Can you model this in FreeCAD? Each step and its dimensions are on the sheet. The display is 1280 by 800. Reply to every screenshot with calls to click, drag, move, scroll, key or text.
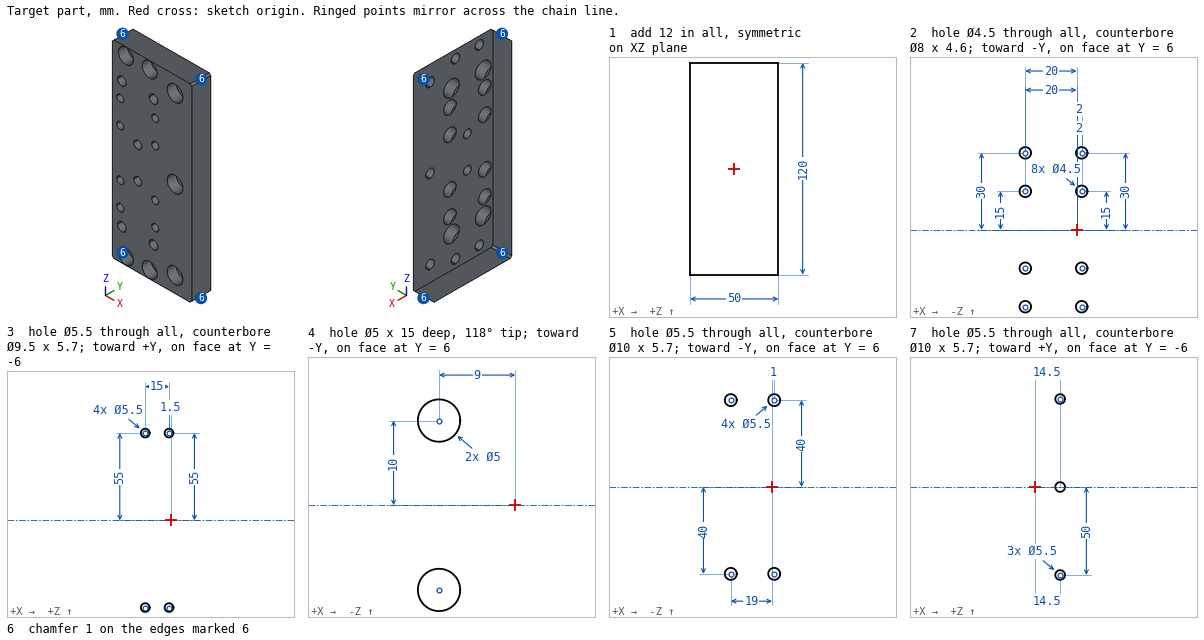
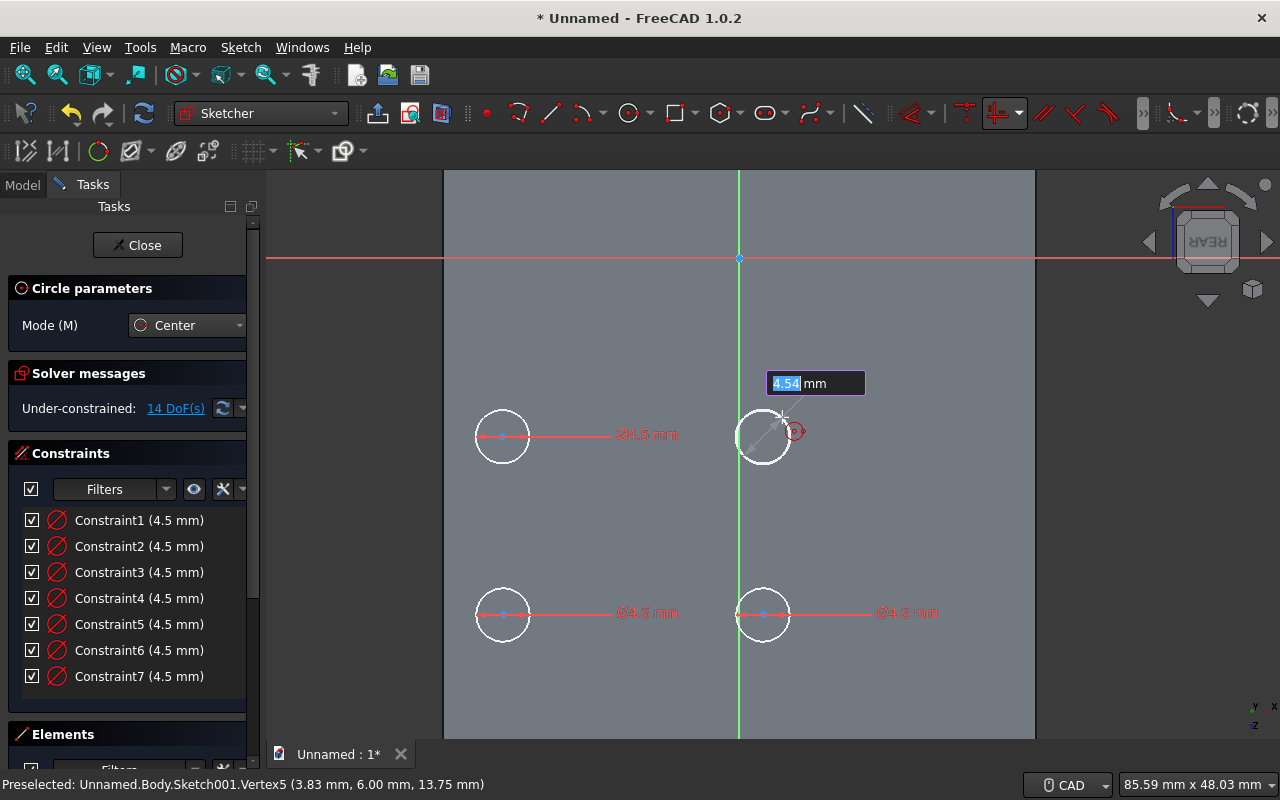
text(4.5)
key(Return)
key(Escape)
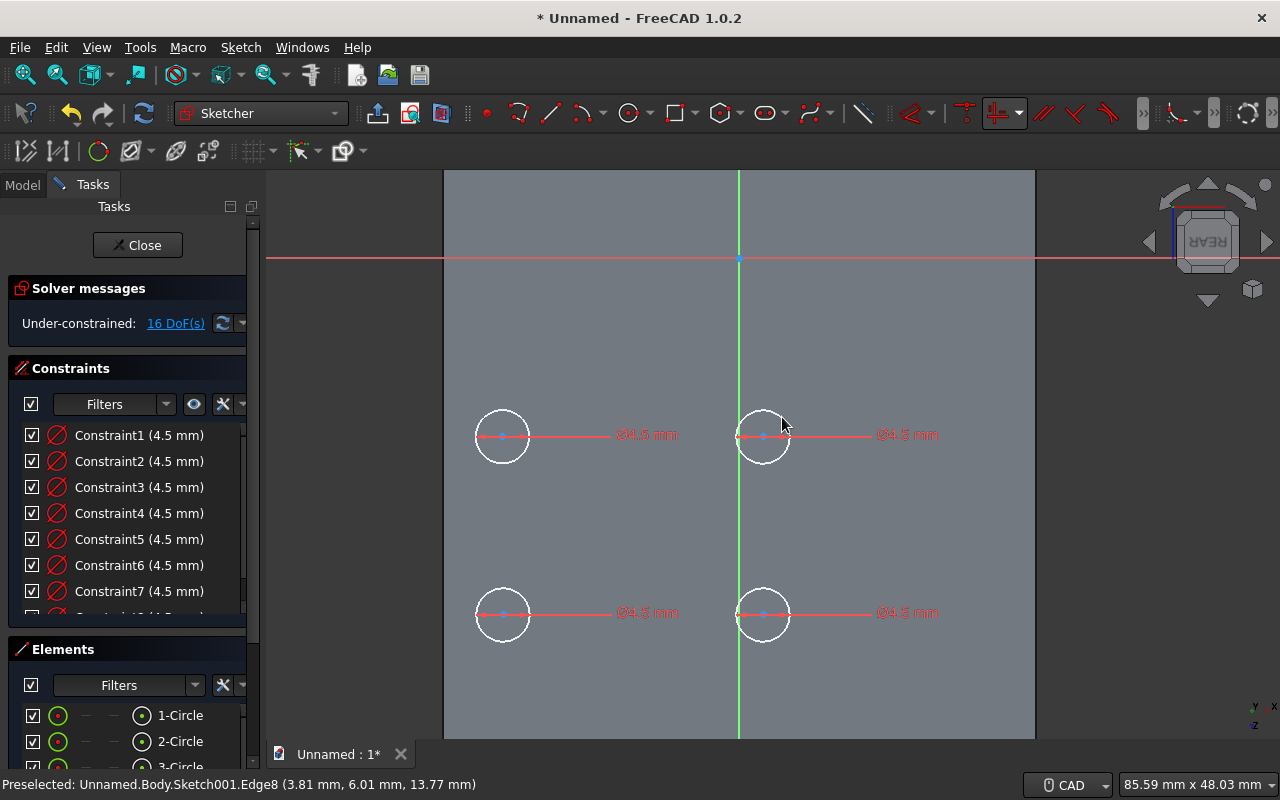
scroll(763, 615, down, 4)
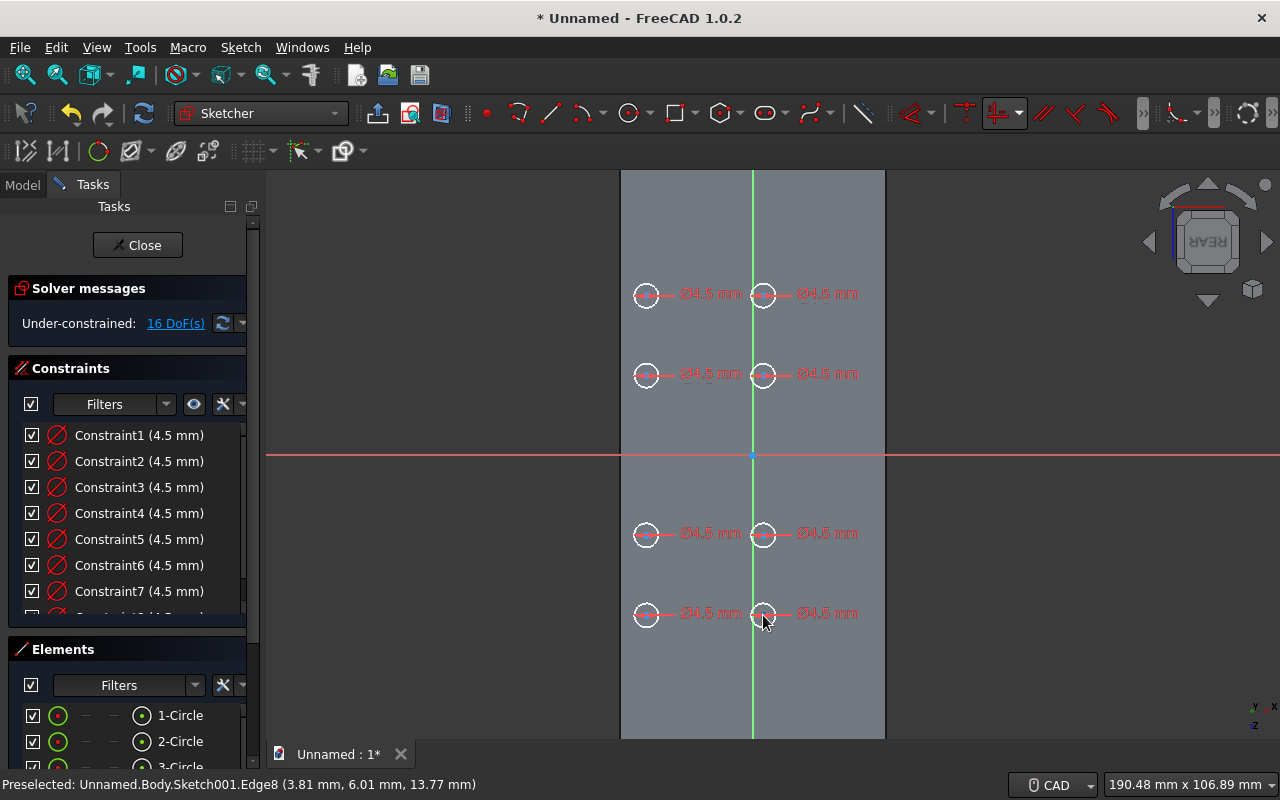
click(646, 376)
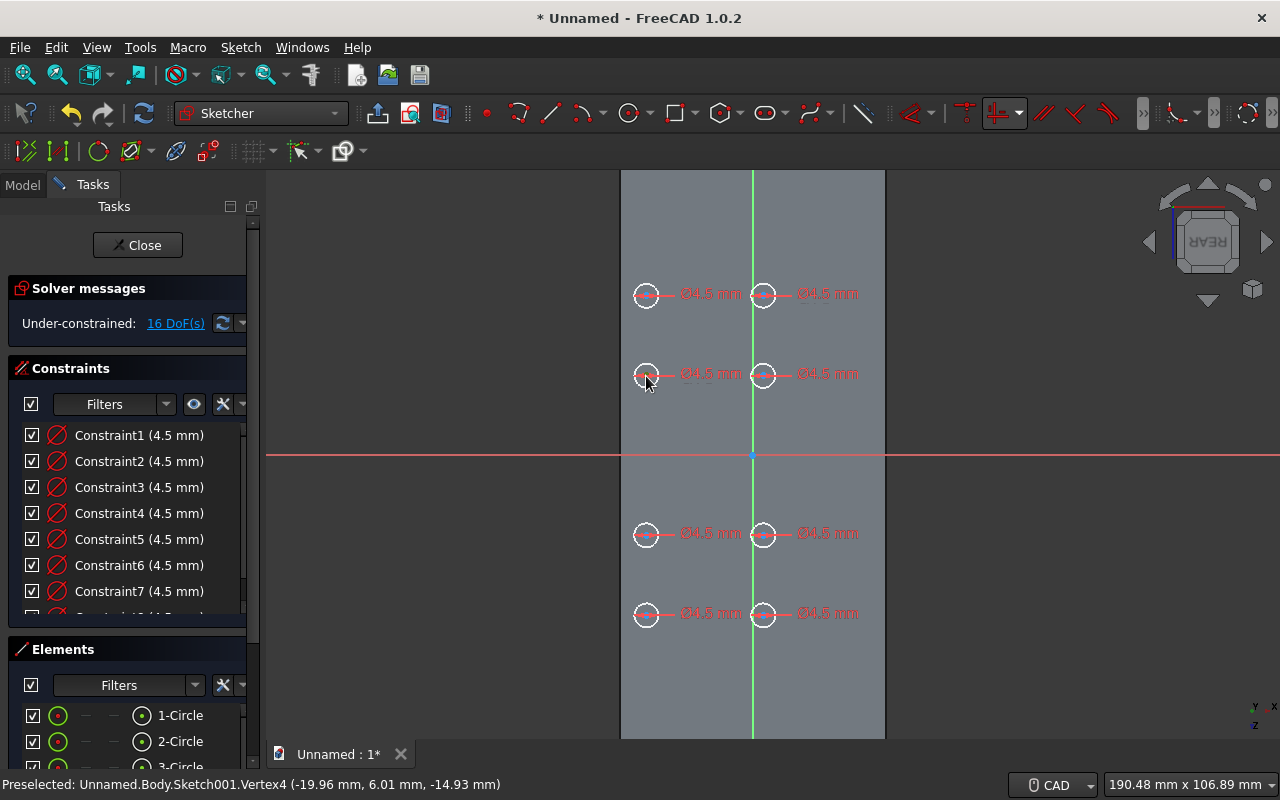
click(646, 535)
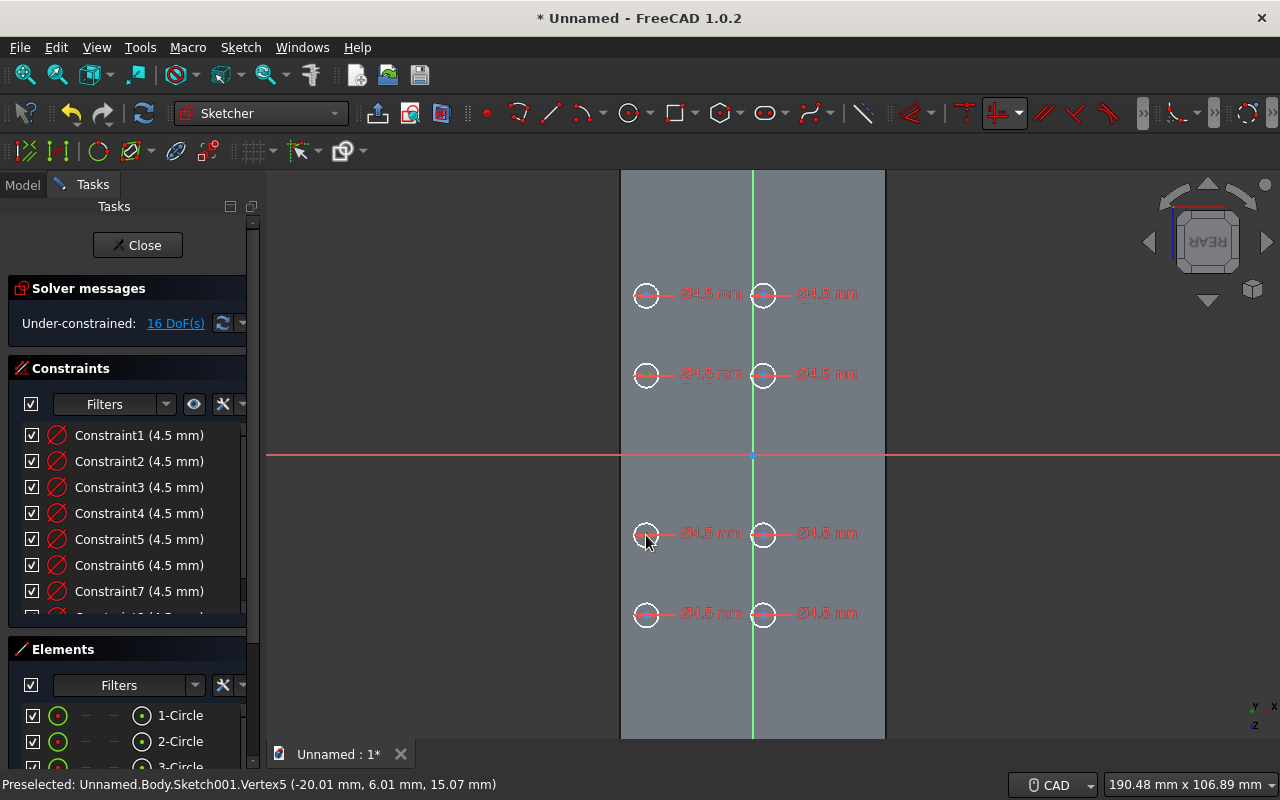
click(353, 455)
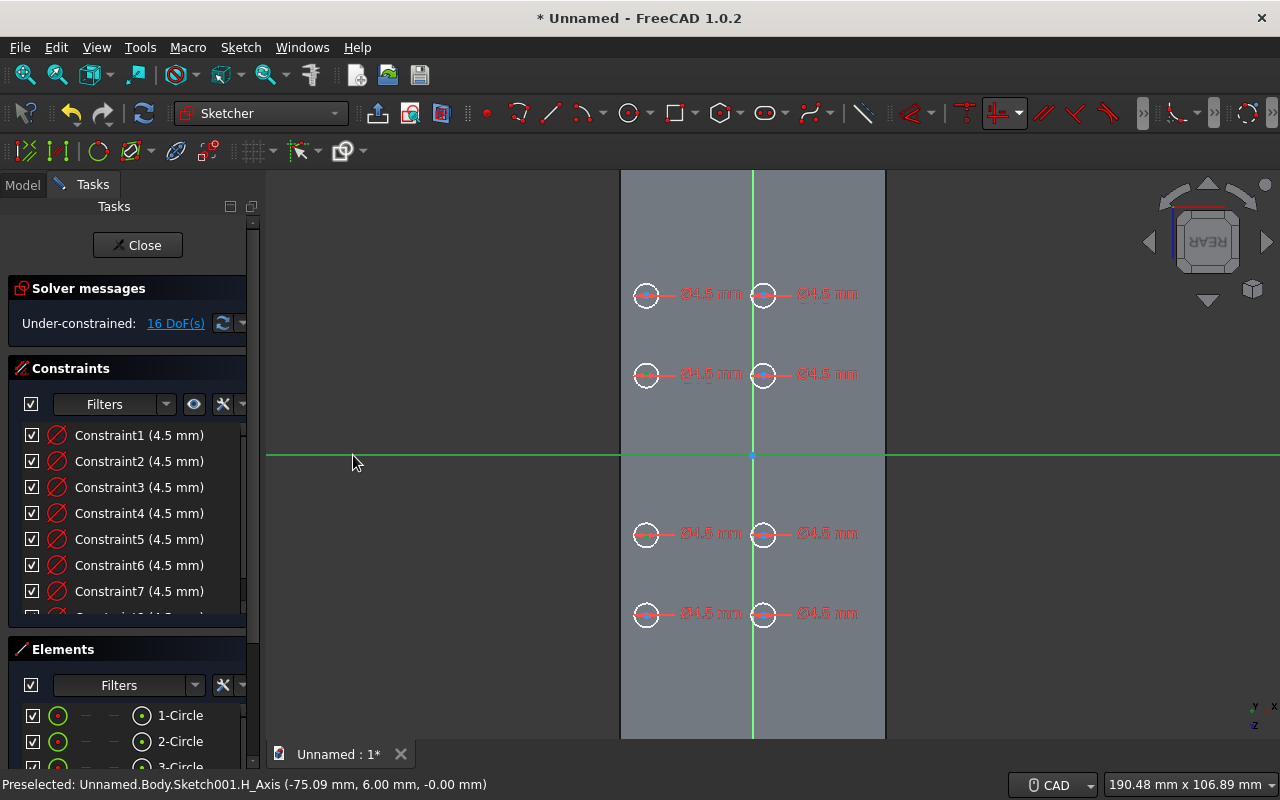
key(s)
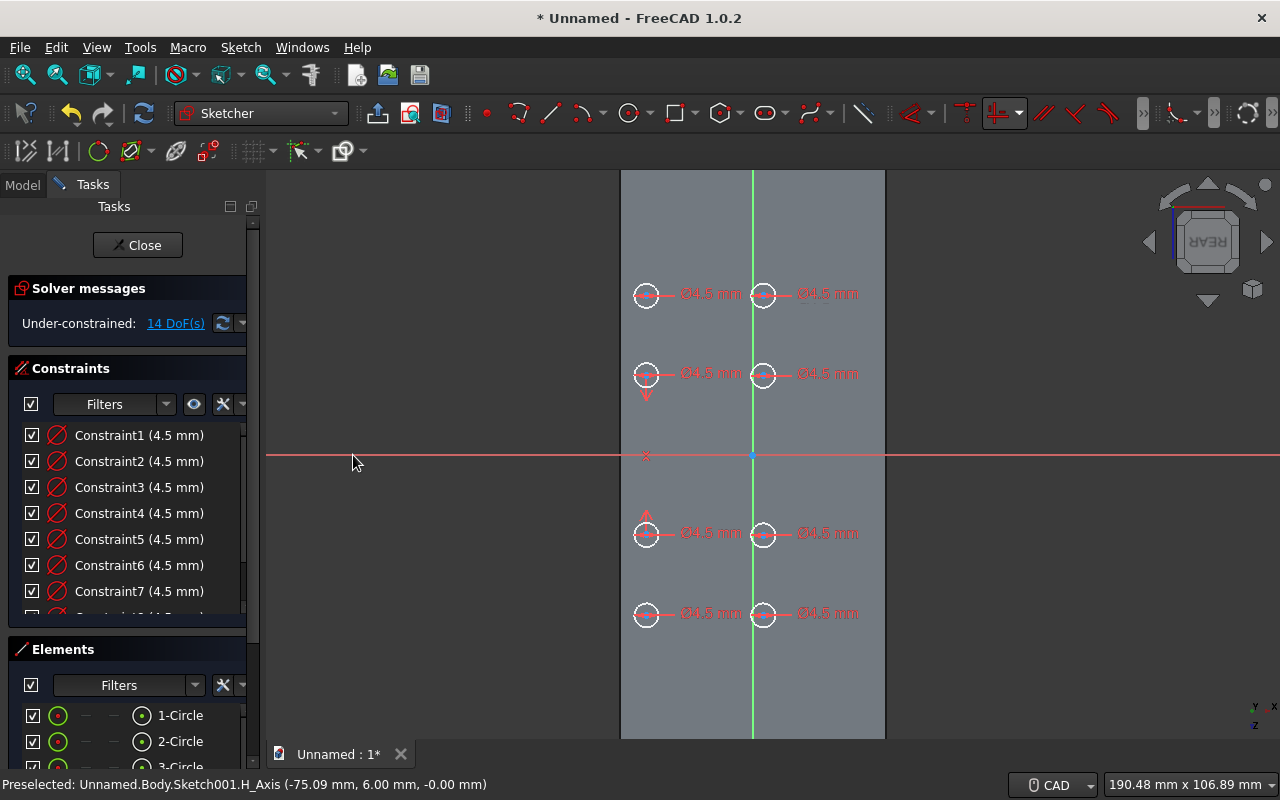
click(763, 296)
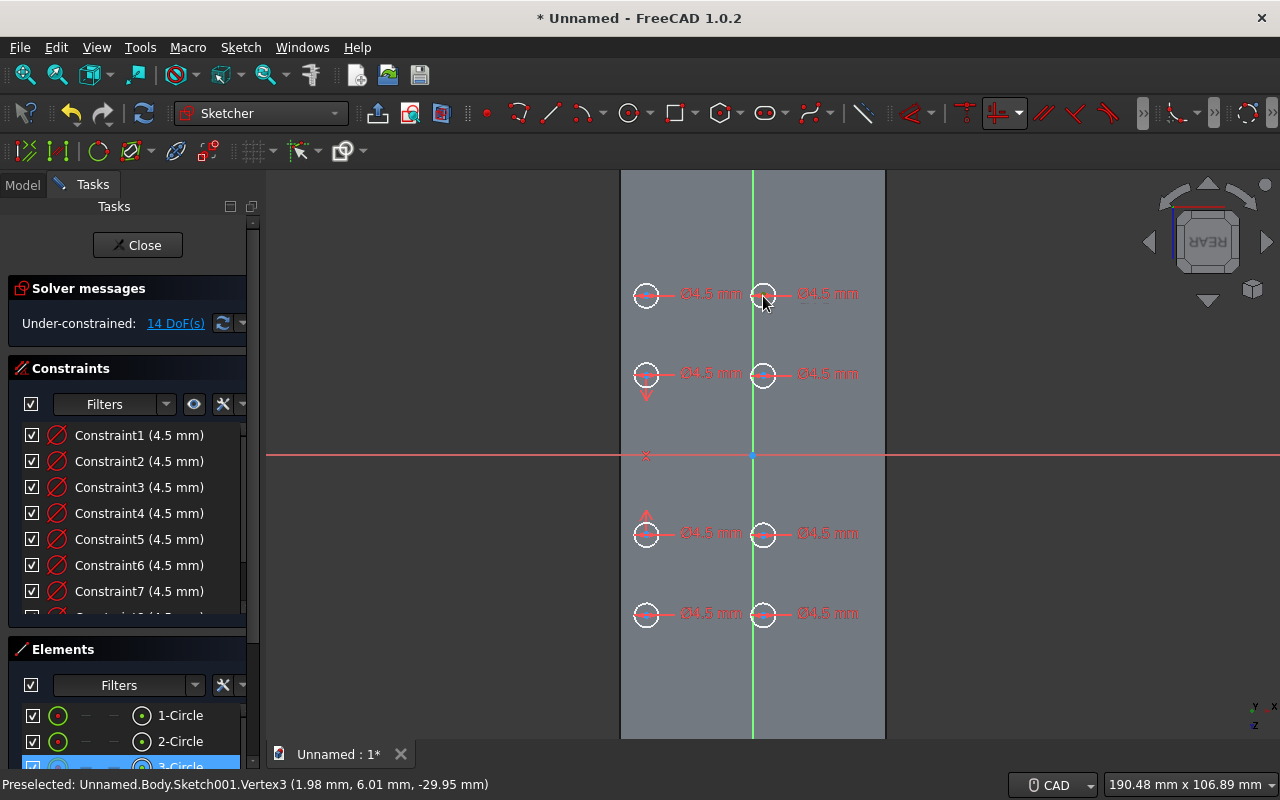
click(763, 615)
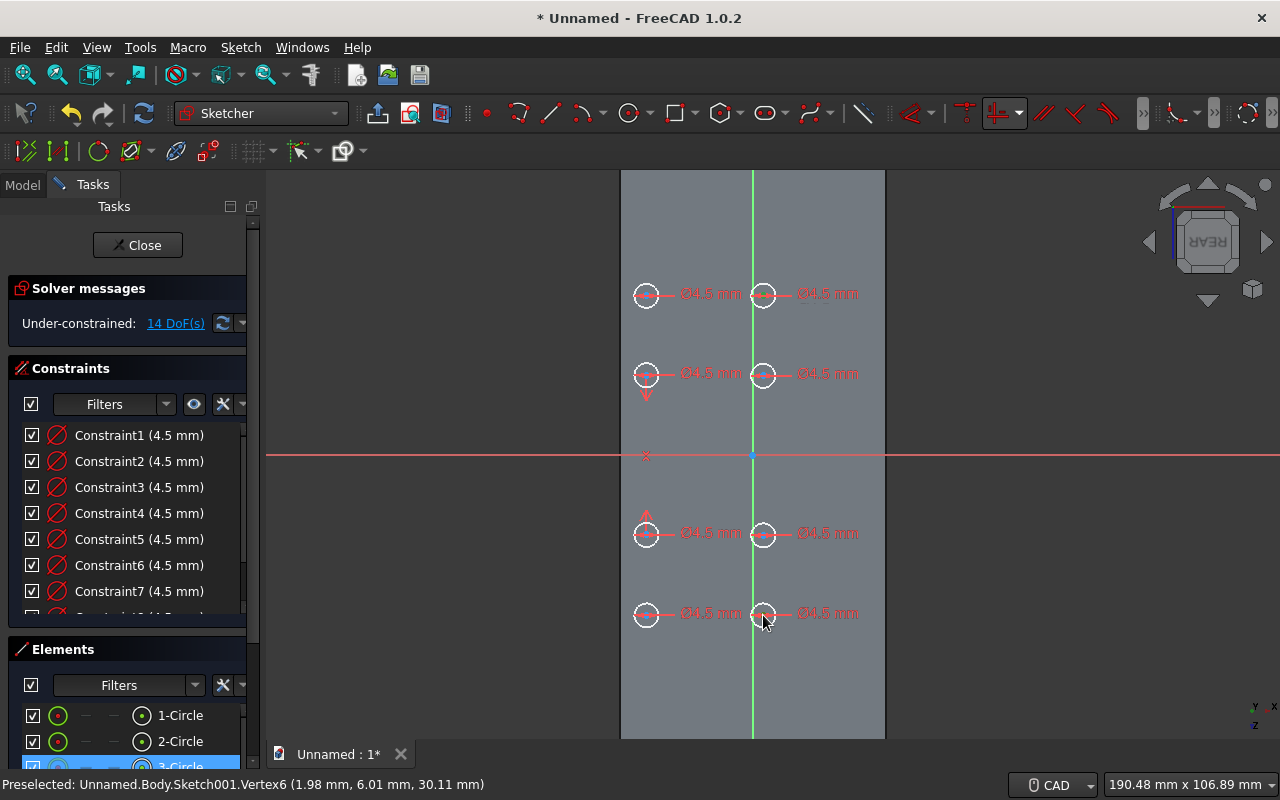
click(353, 455)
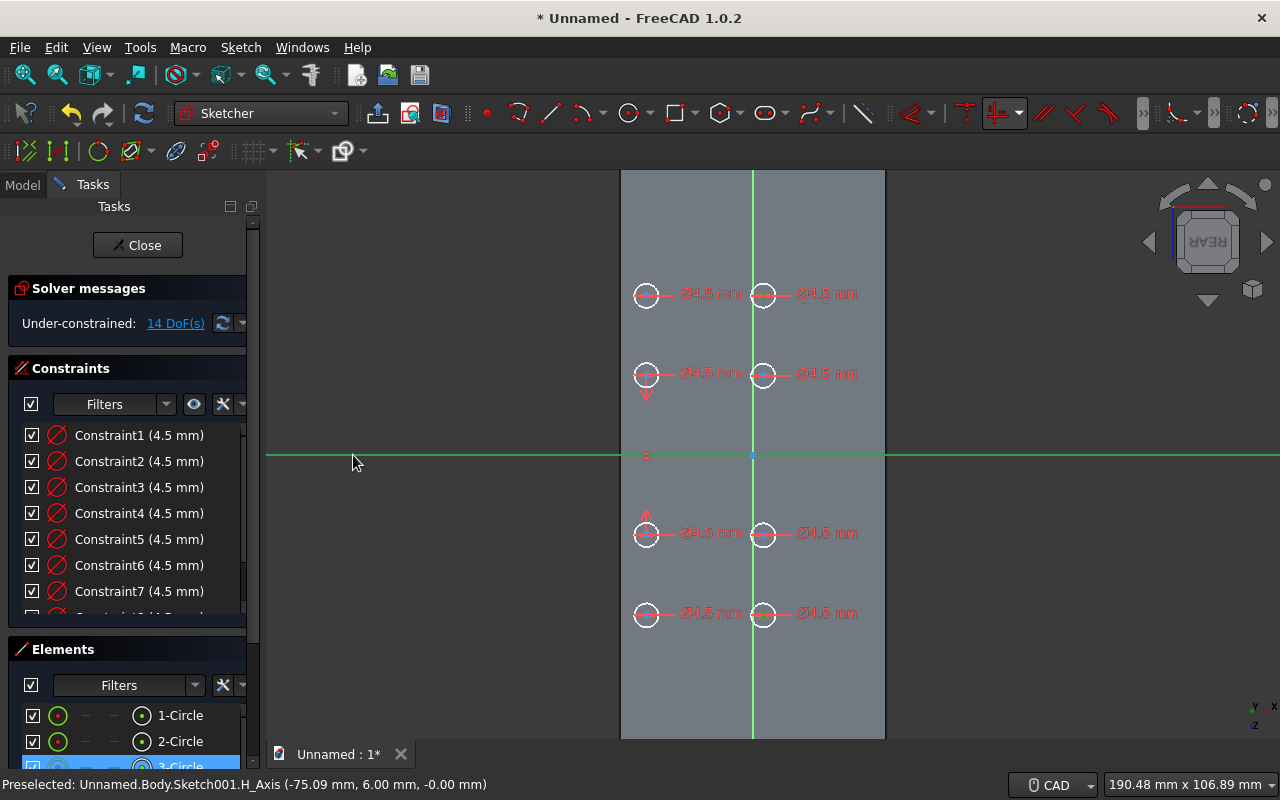
key(s)